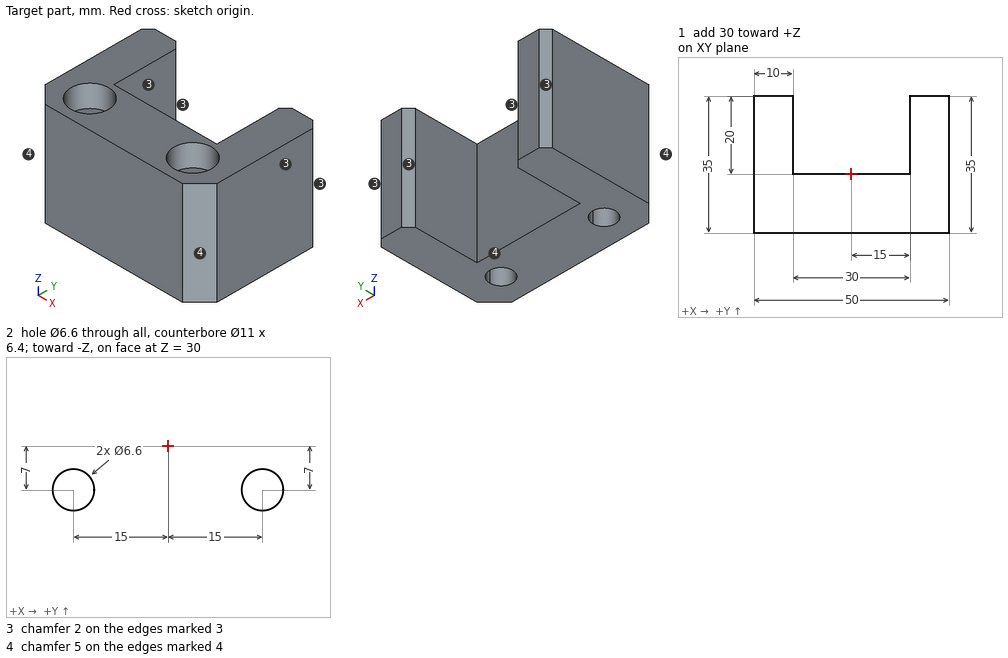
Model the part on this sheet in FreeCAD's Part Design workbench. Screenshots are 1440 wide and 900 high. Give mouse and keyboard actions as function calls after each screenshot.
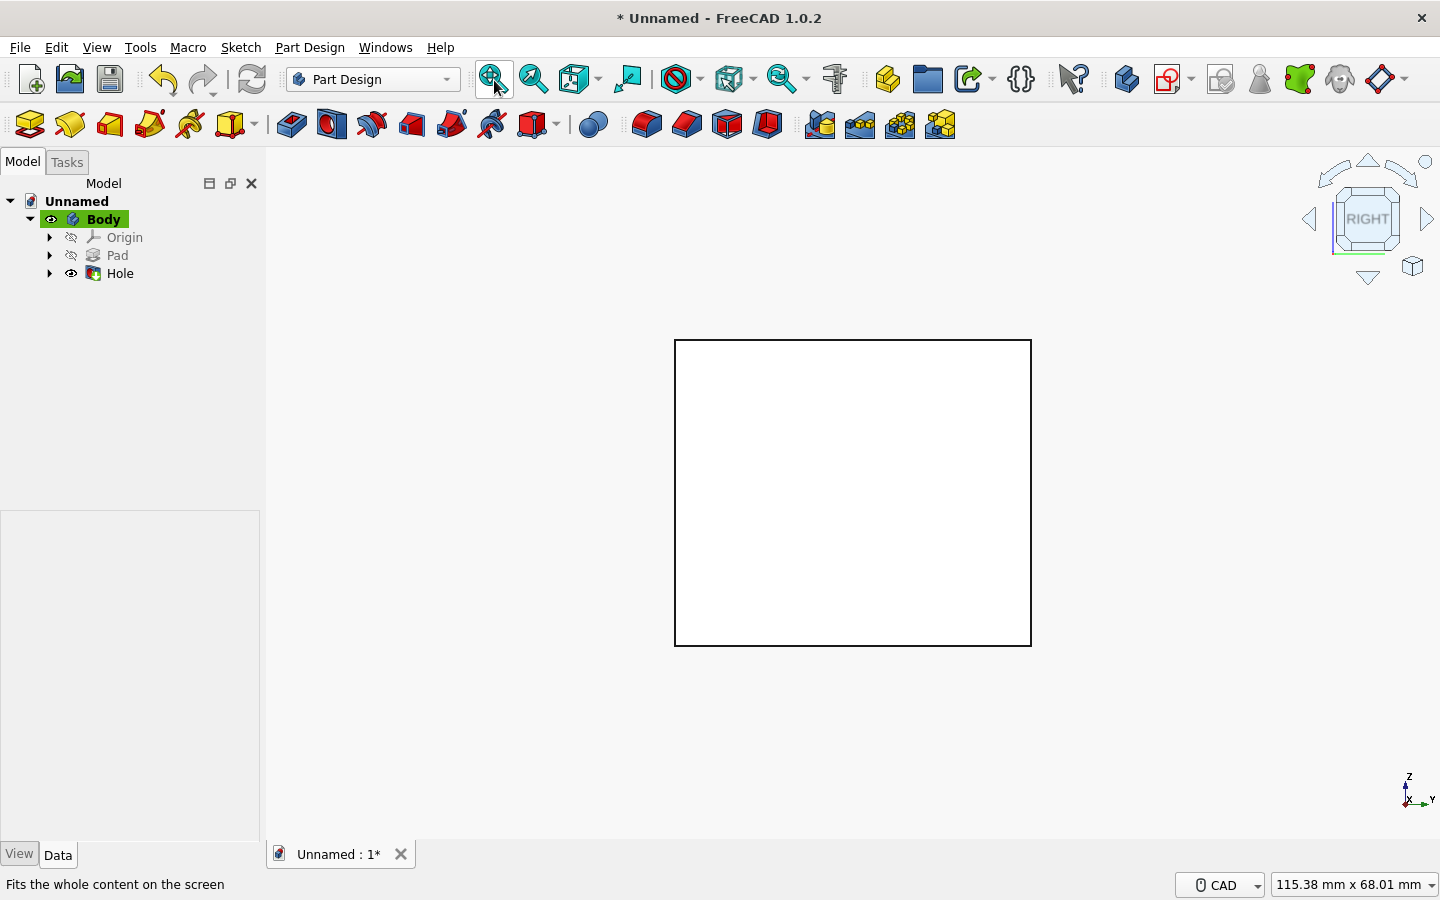
click(494, 80)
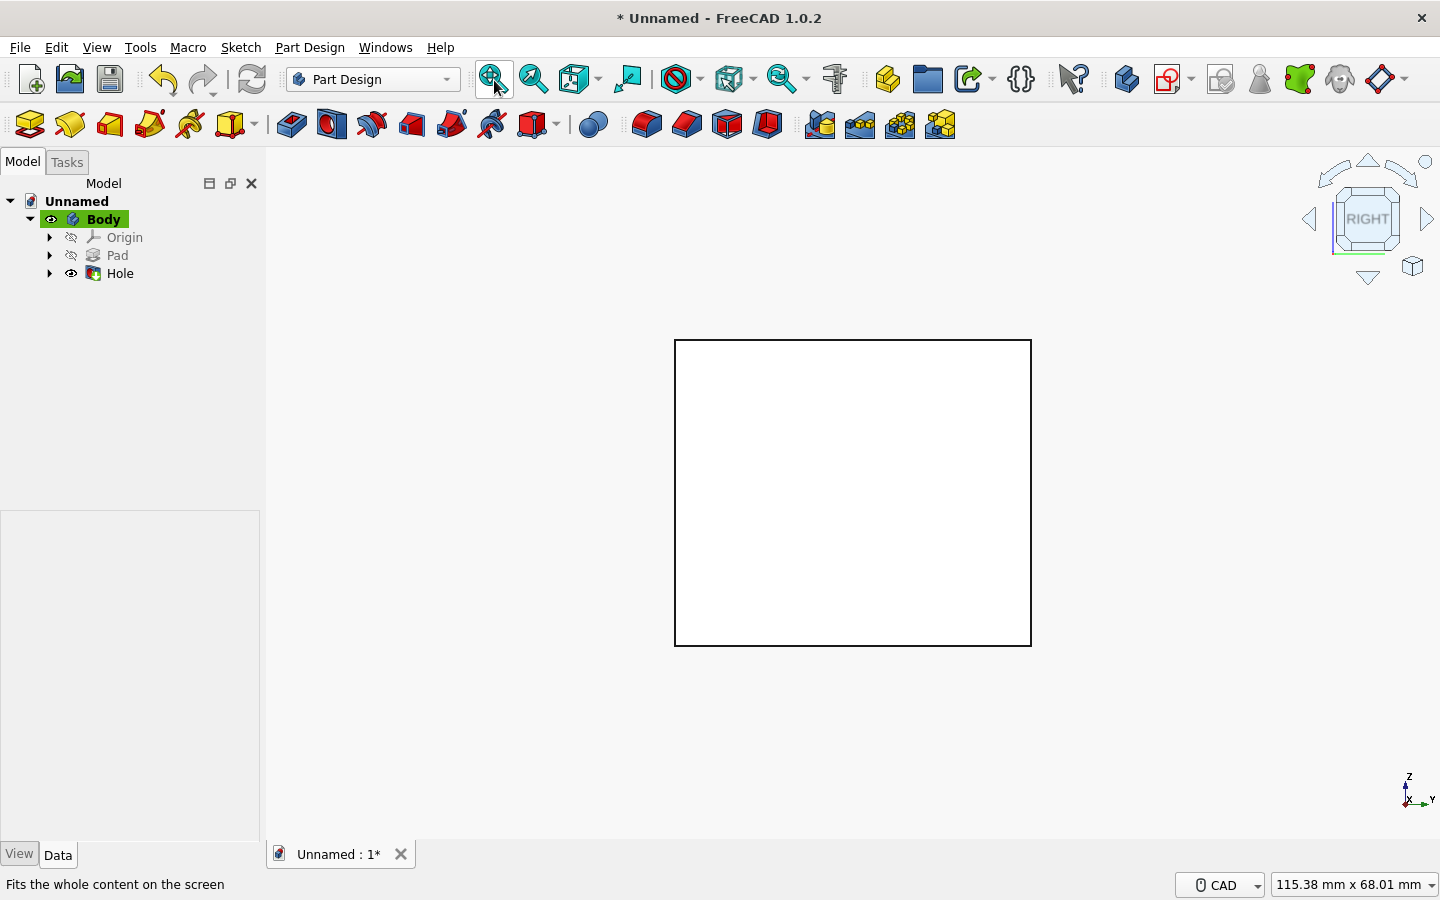
click(1031, 492)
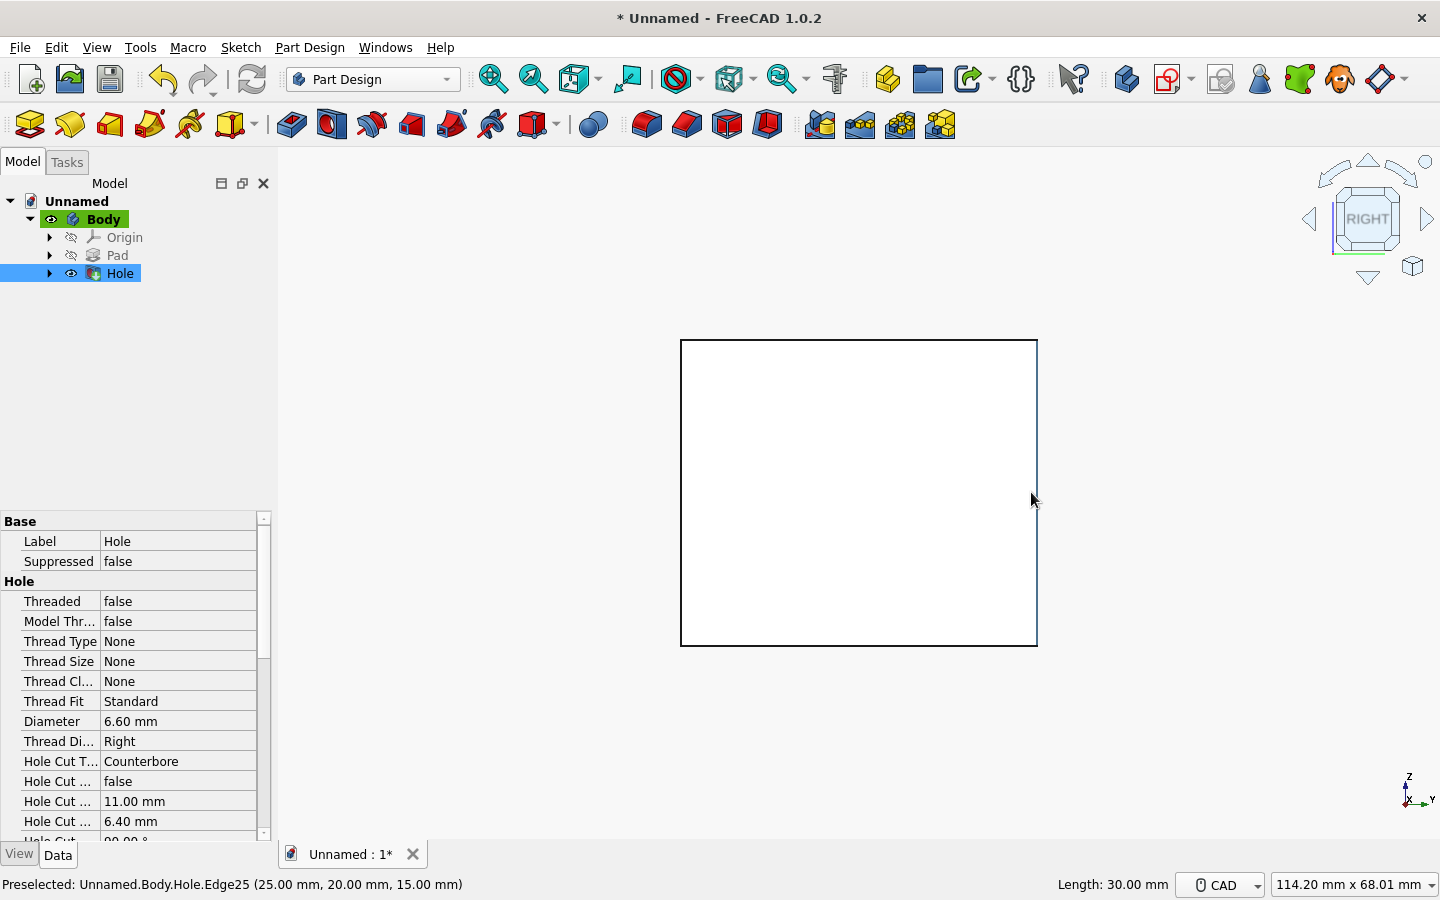
key(5)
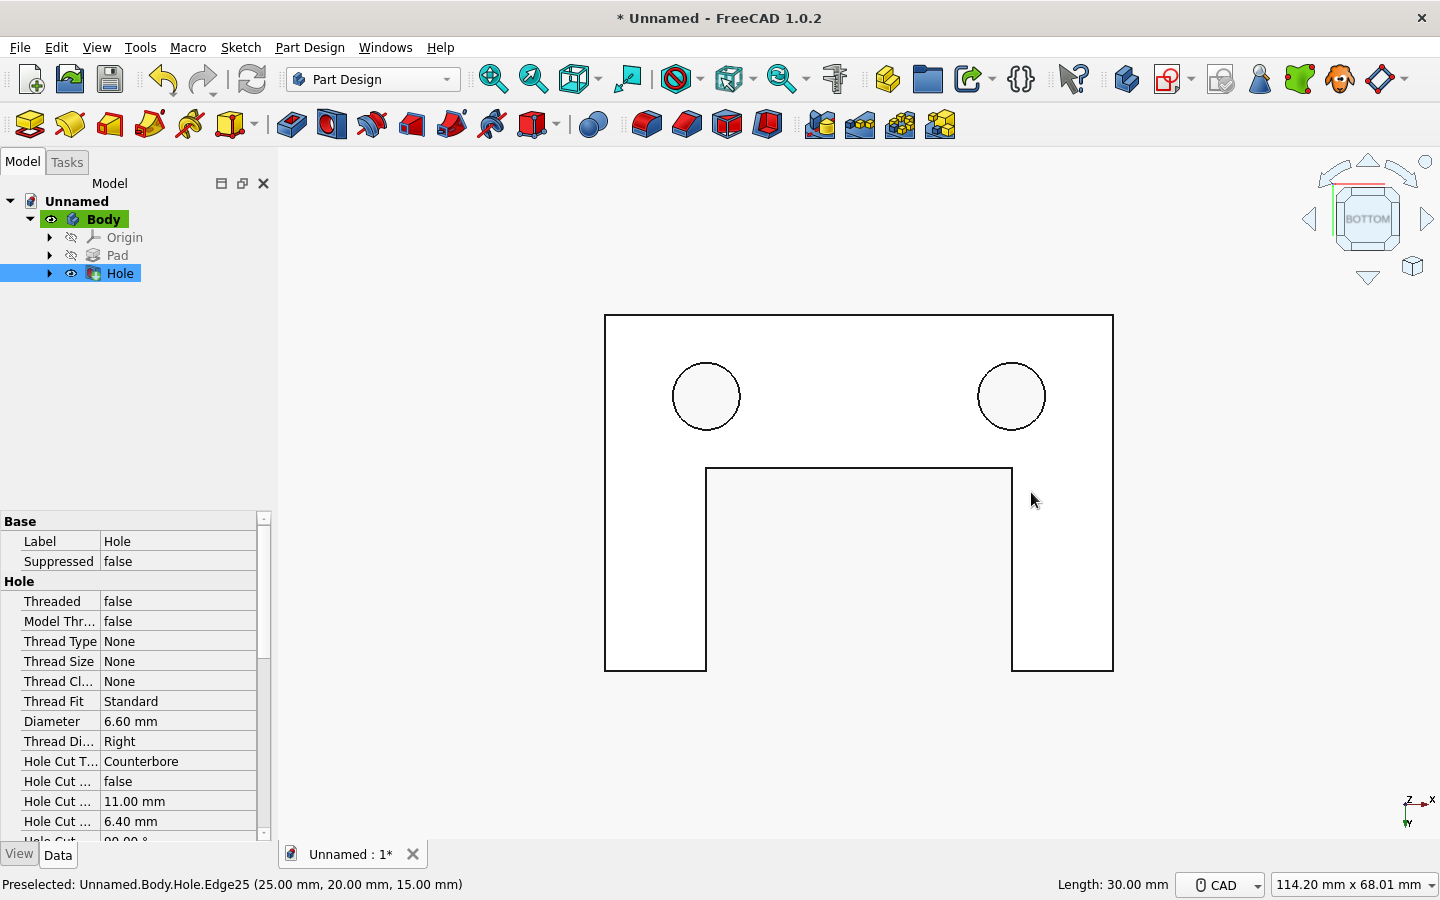
key(4)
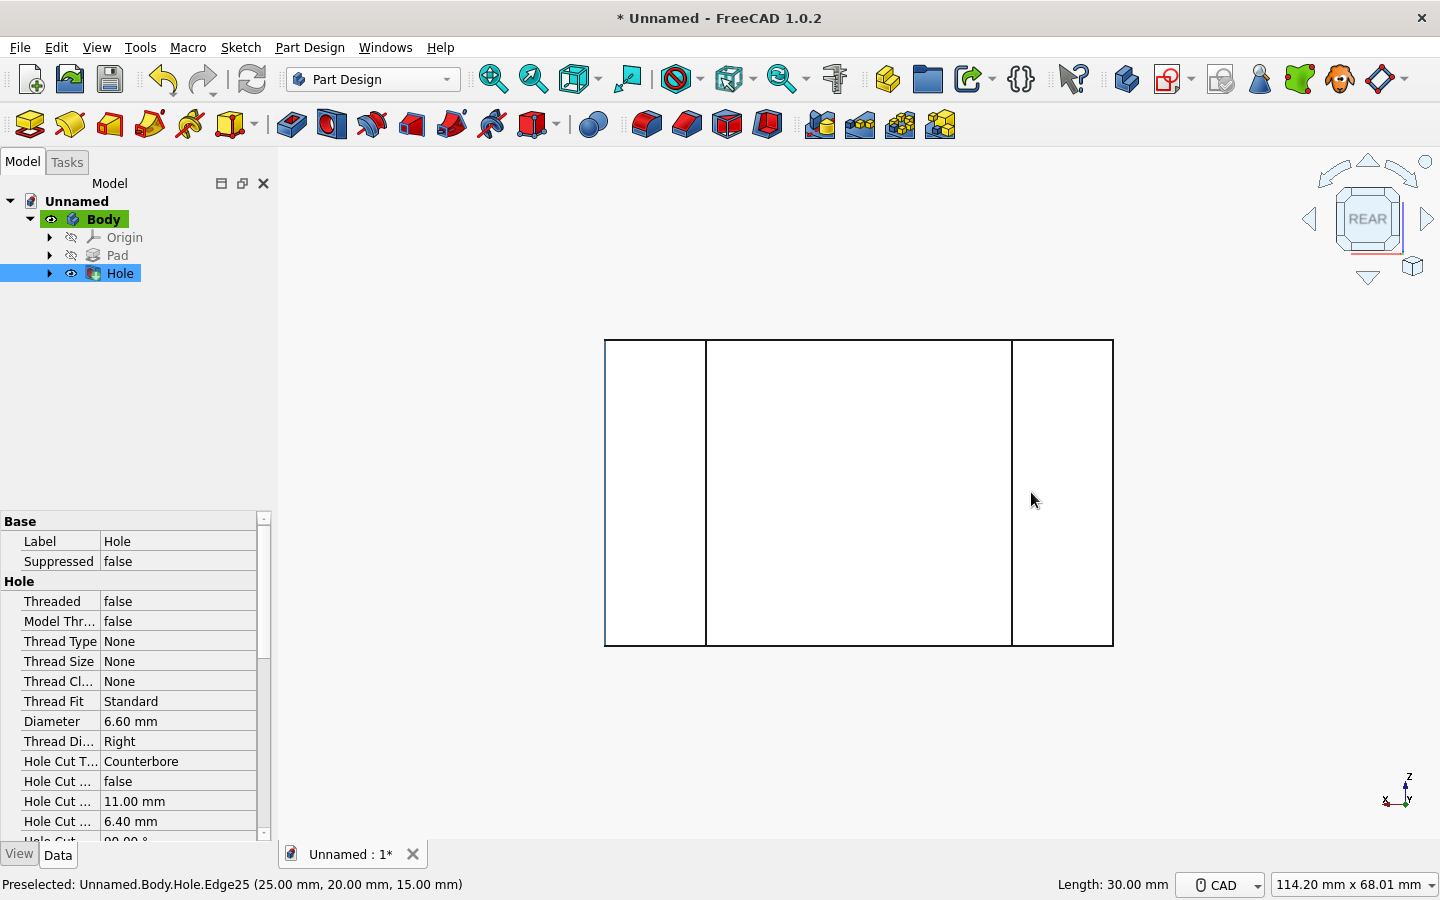
click(494, 80)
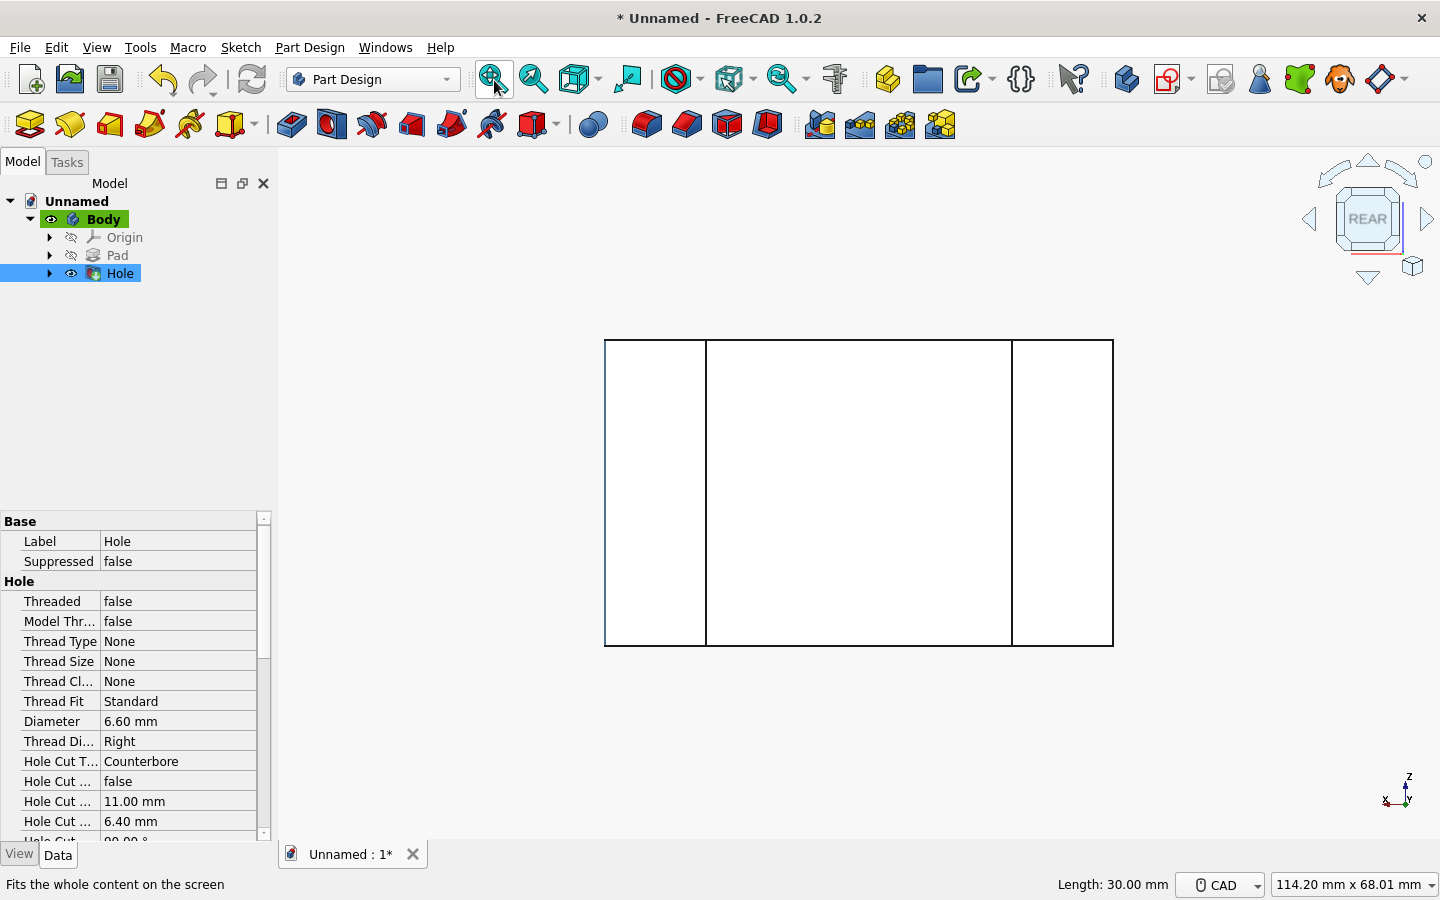
click(1113, 492, ctrl)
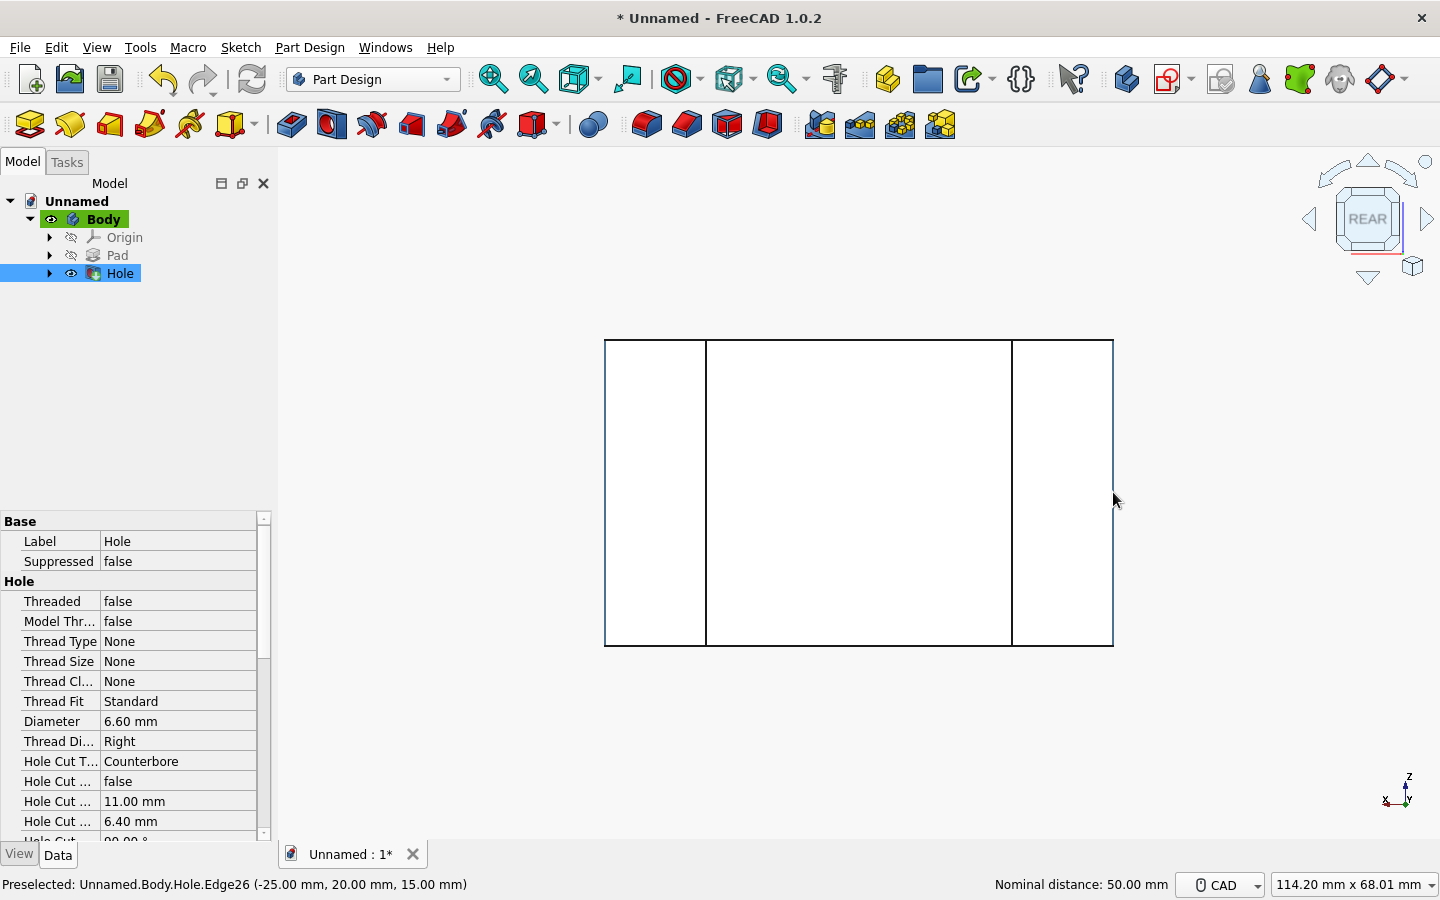
click(1012, 492, ctrl)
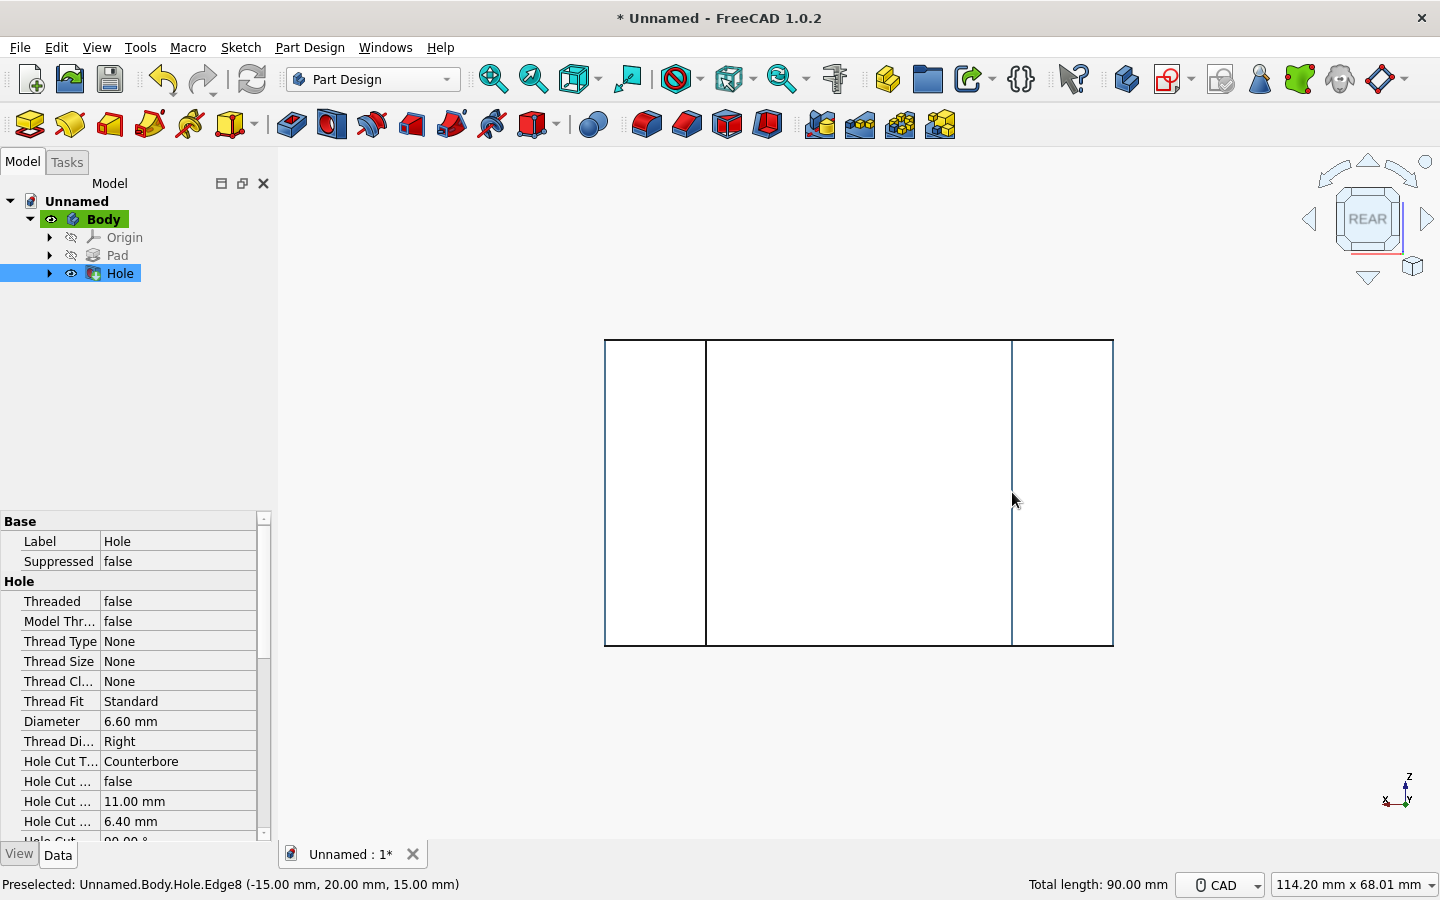
click(706, 492, ctrl)